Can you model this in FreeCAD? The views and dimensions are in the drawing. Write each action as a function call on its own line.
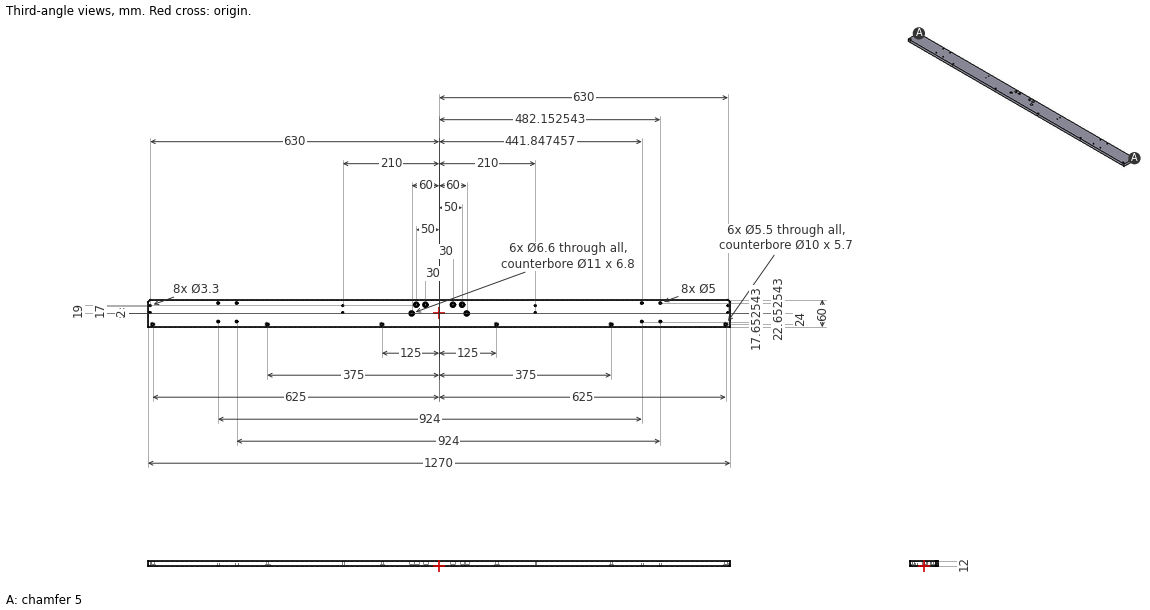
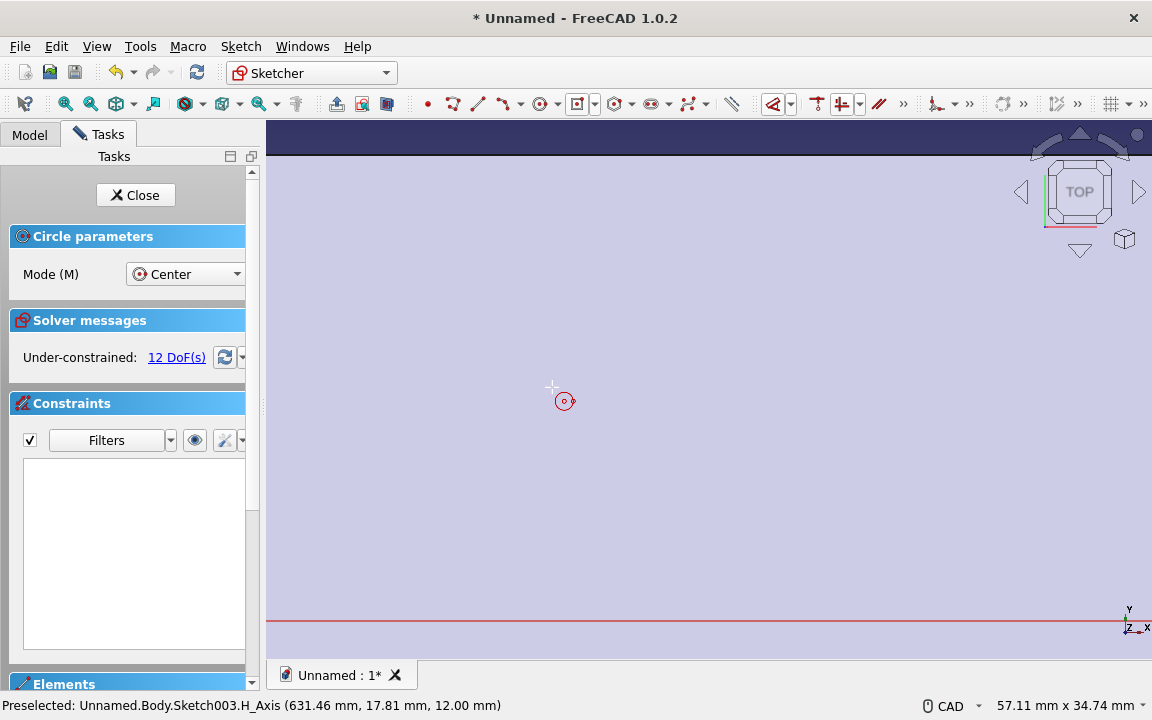
scroll(552, 387, down, 18)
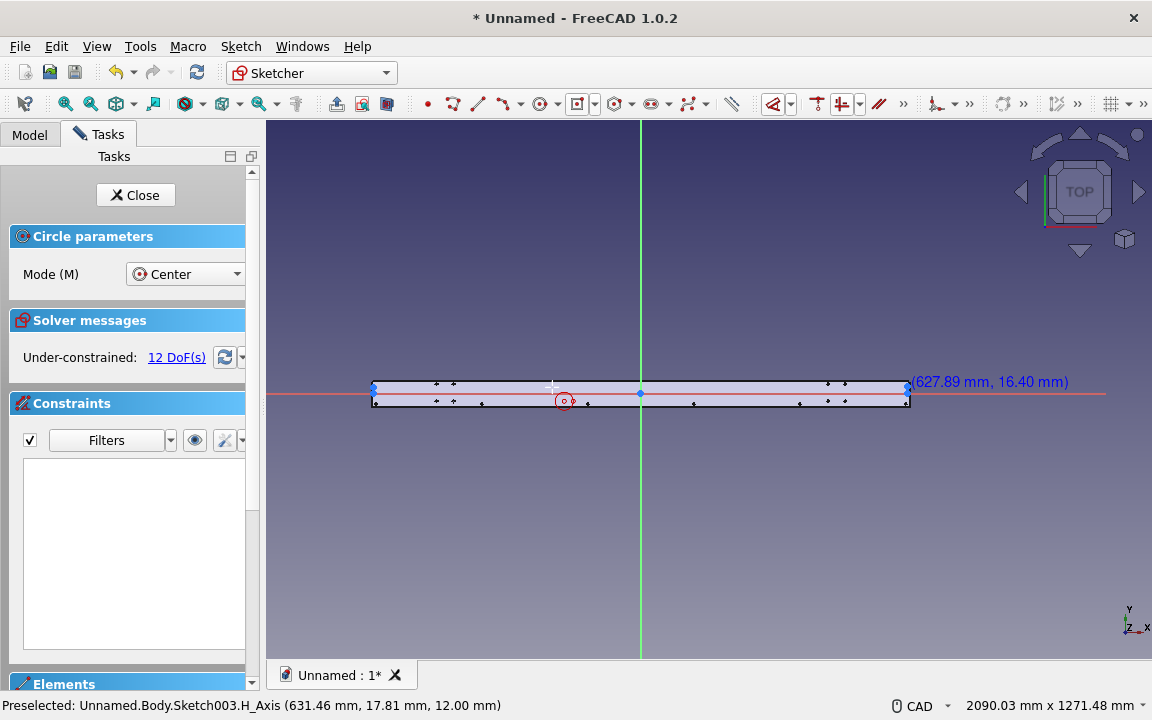
scroll(552, 387, up, 4)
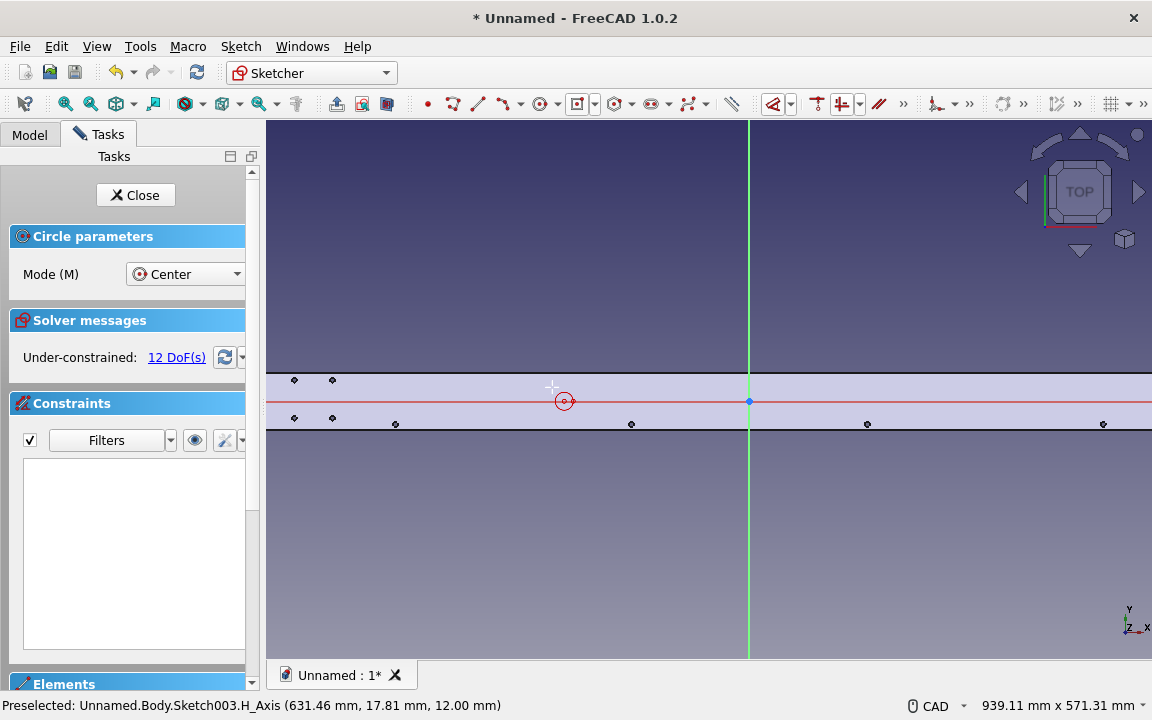
click(551, 386)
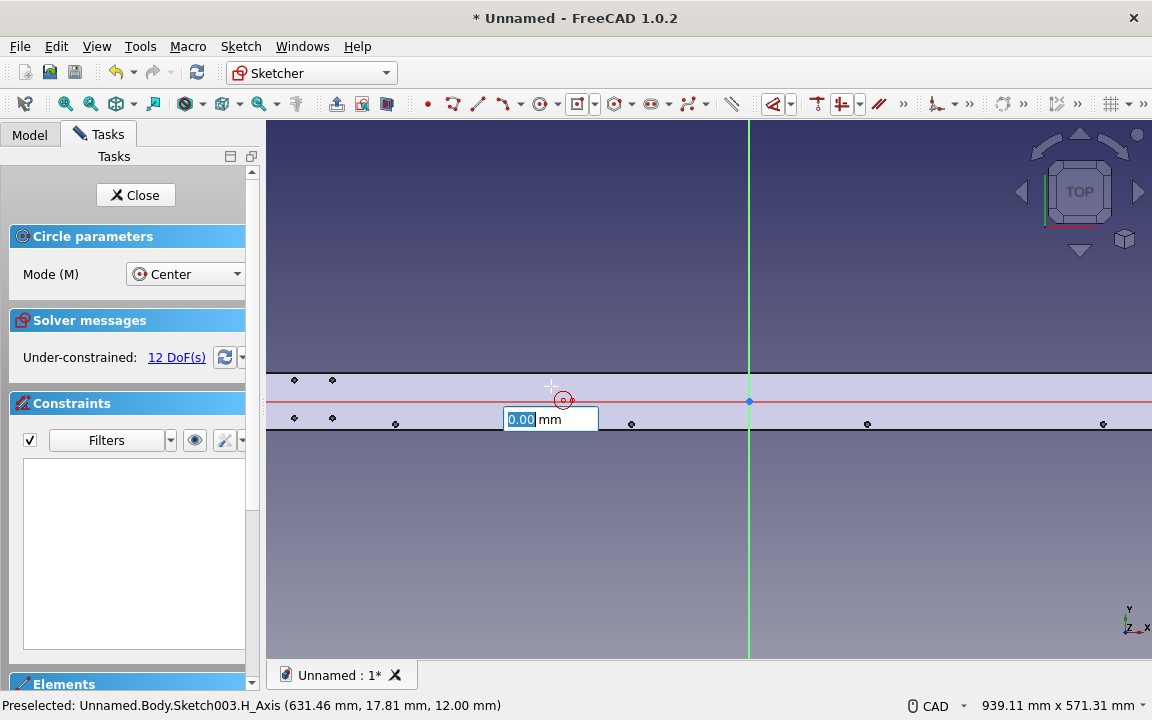
scroll(552, 385, up, 12)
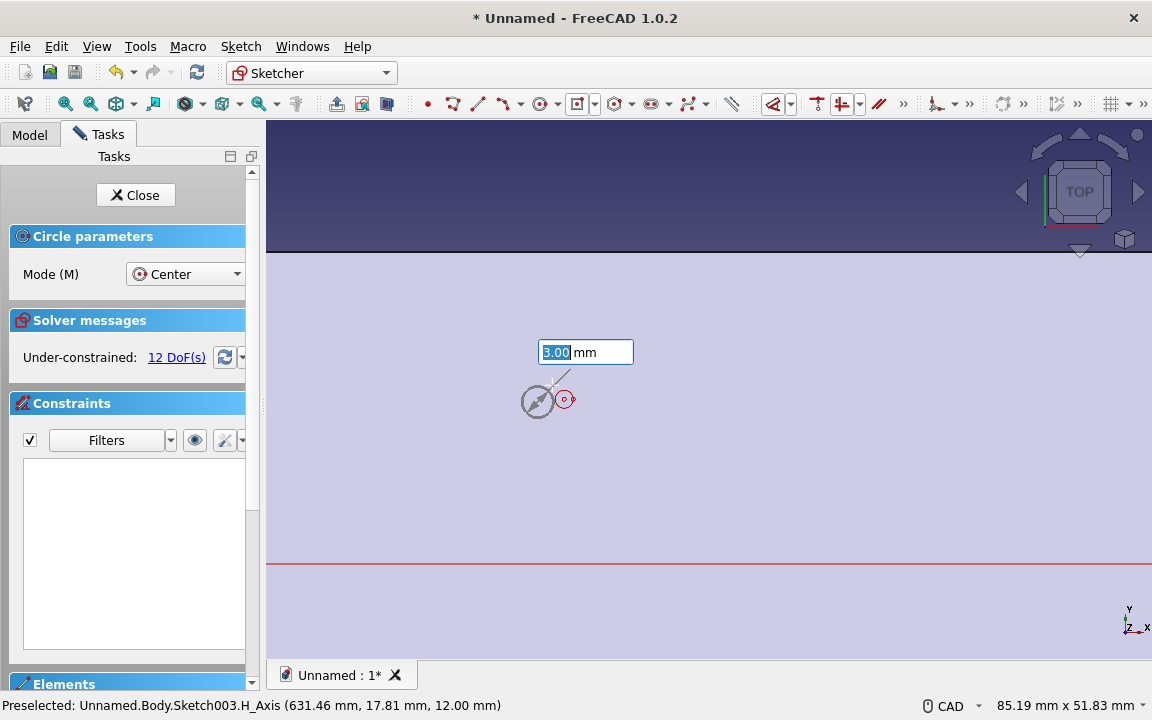
click(552, 375)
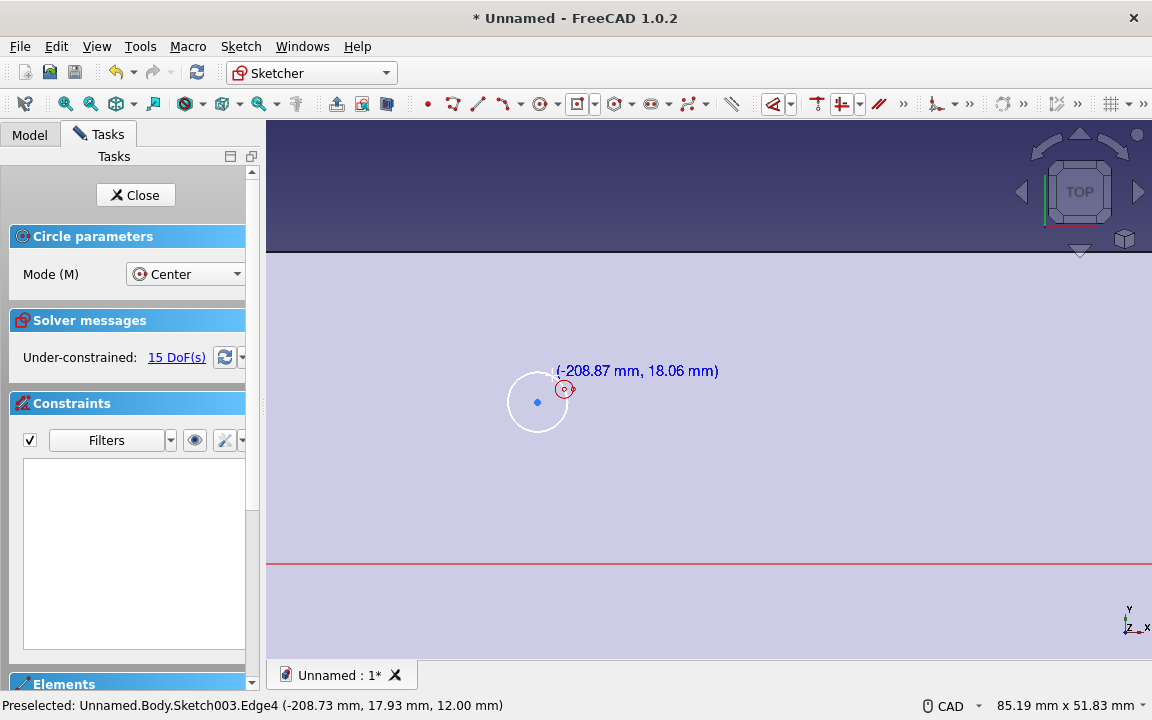
scroll(540, 543, up, 2)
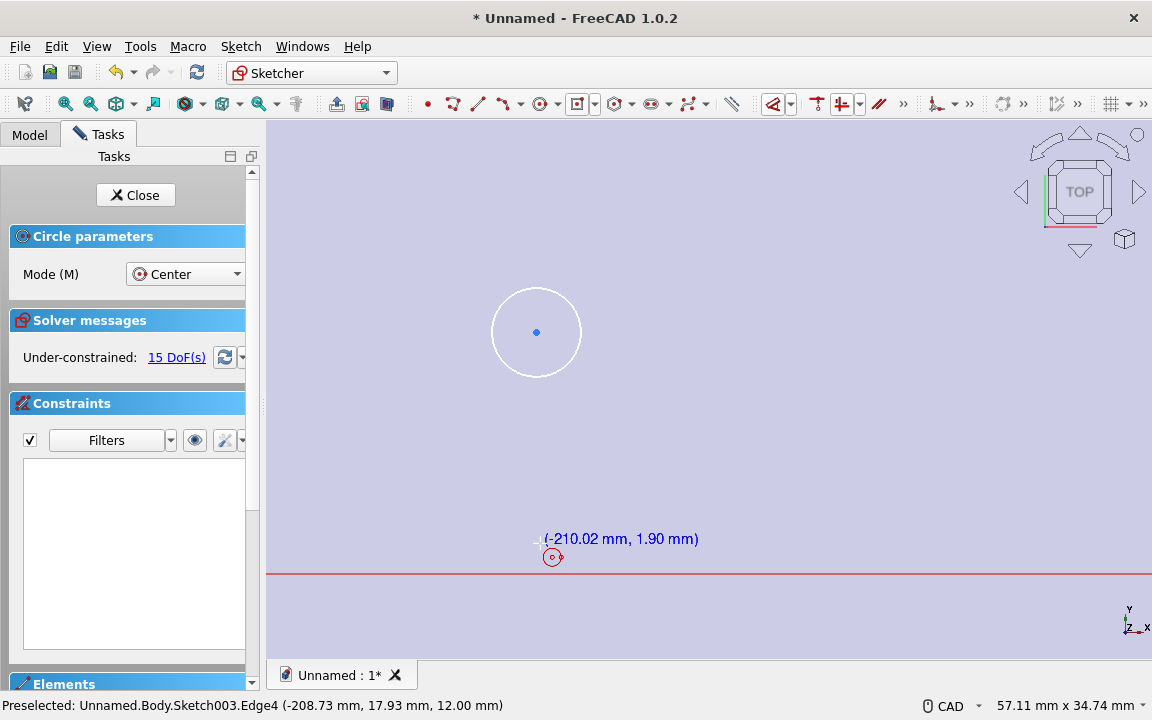
click(540, 543)
click(558, 524)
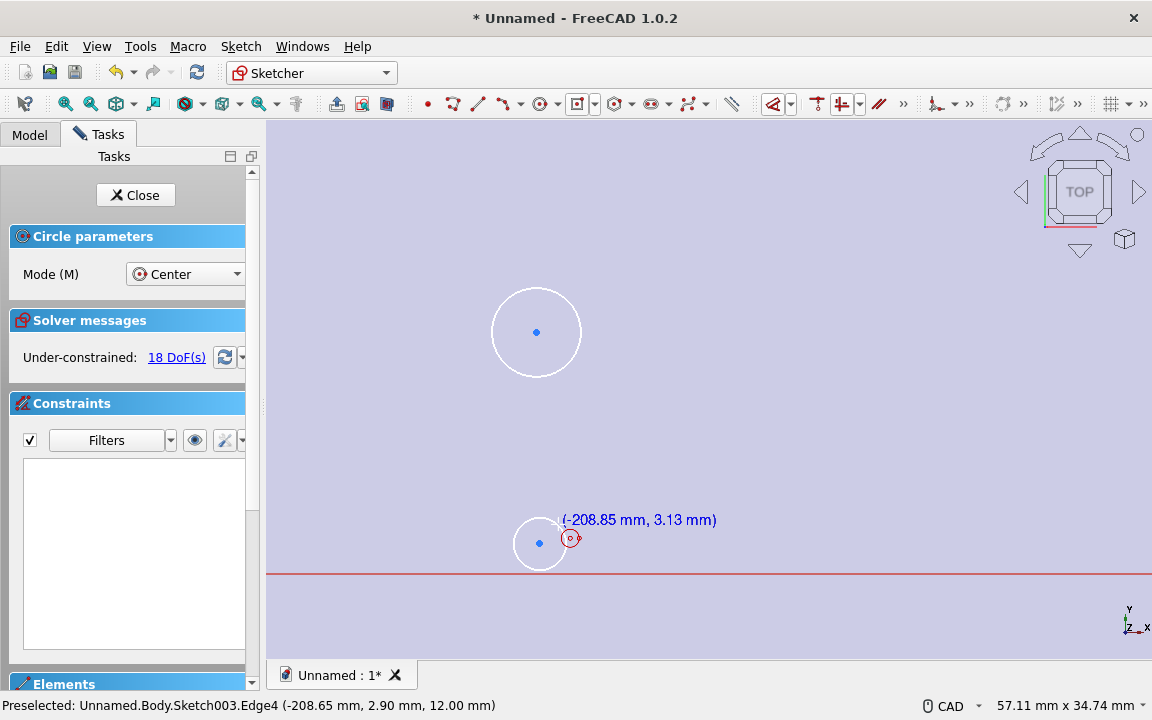
scroll(552, 388, down, 18)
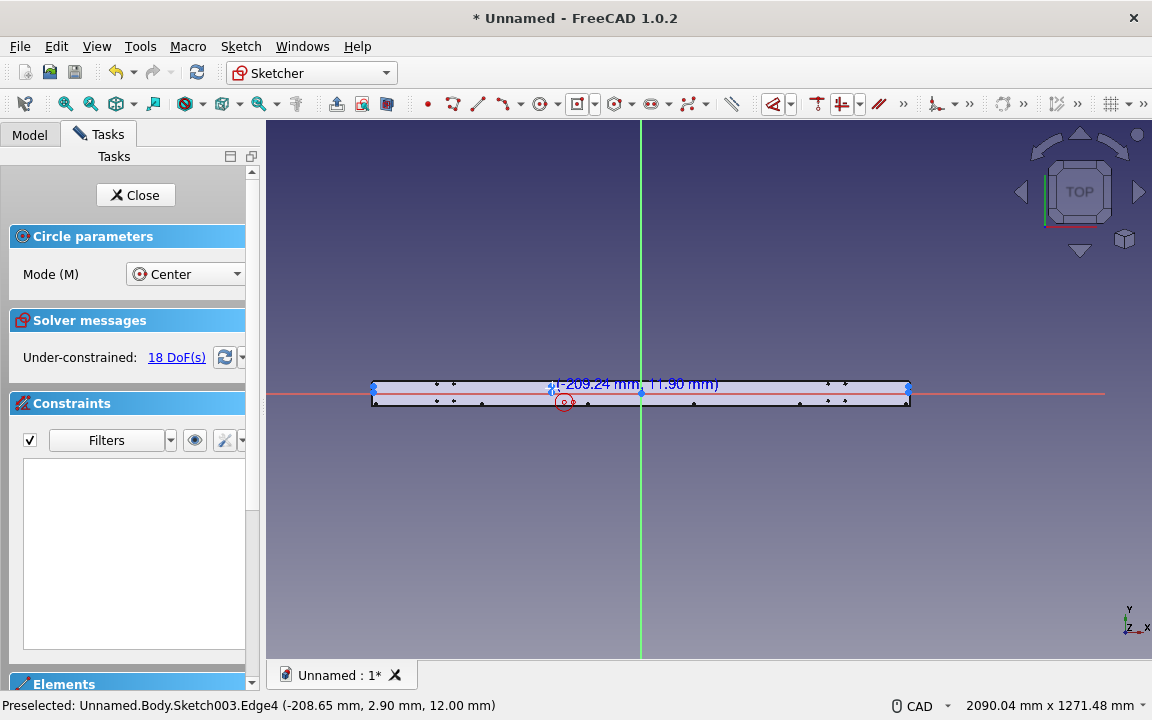
scroll(730, 393, up, 18)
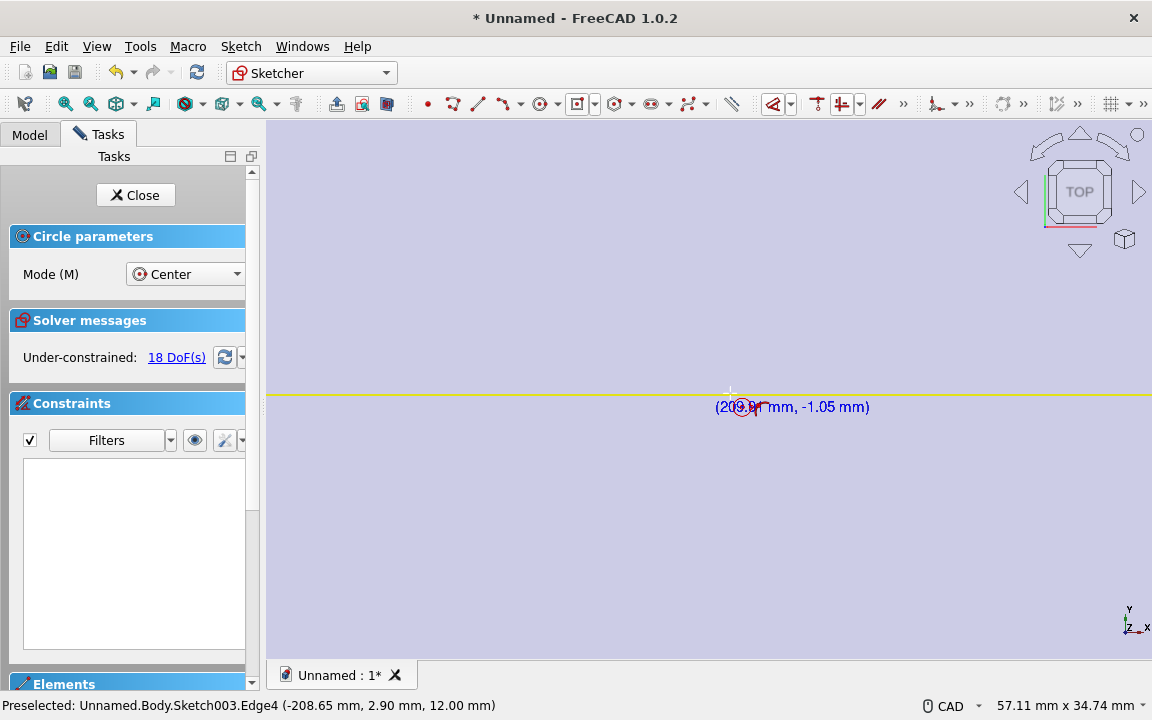
click(713, 364)
click(731, 346)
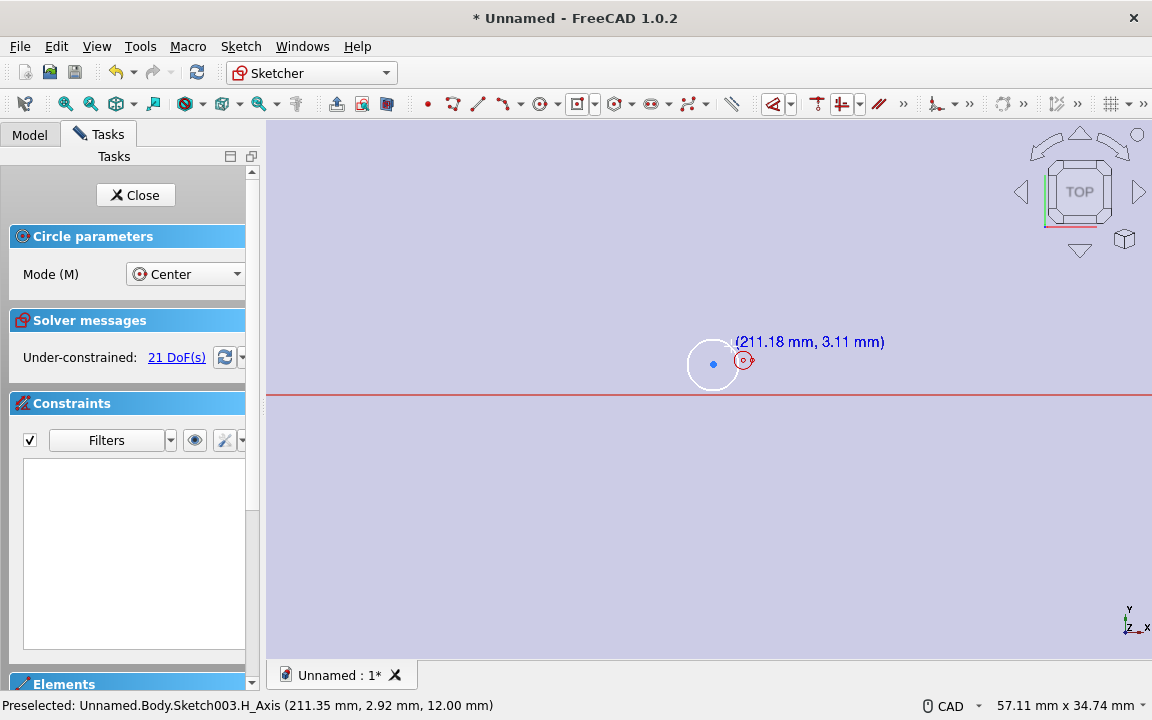
scroll(730, 393, down, 18)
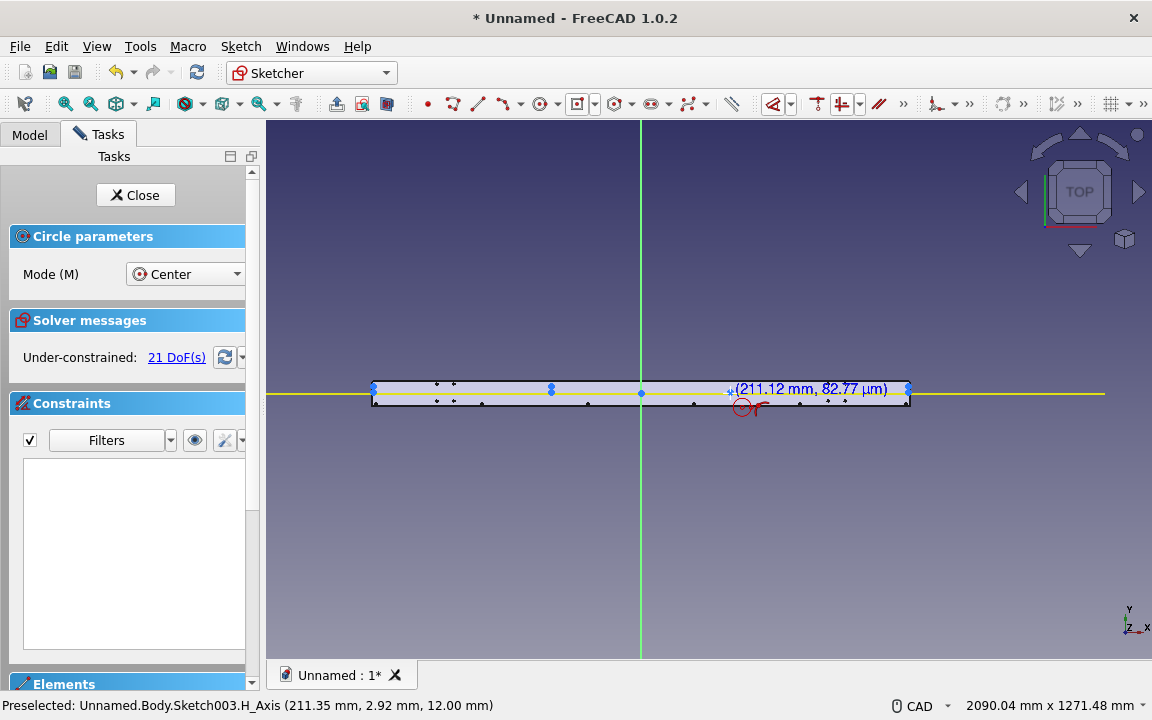
scroll(730, 386, up, 18)